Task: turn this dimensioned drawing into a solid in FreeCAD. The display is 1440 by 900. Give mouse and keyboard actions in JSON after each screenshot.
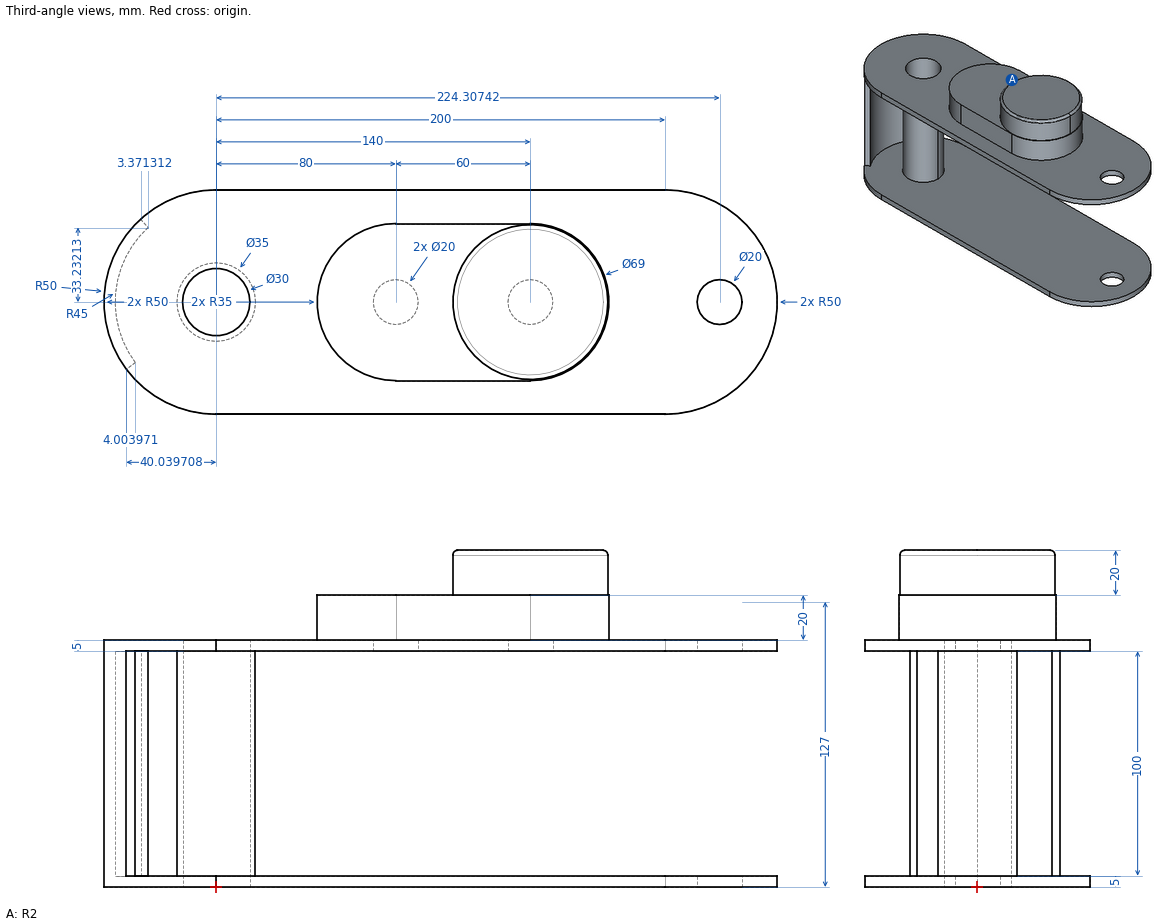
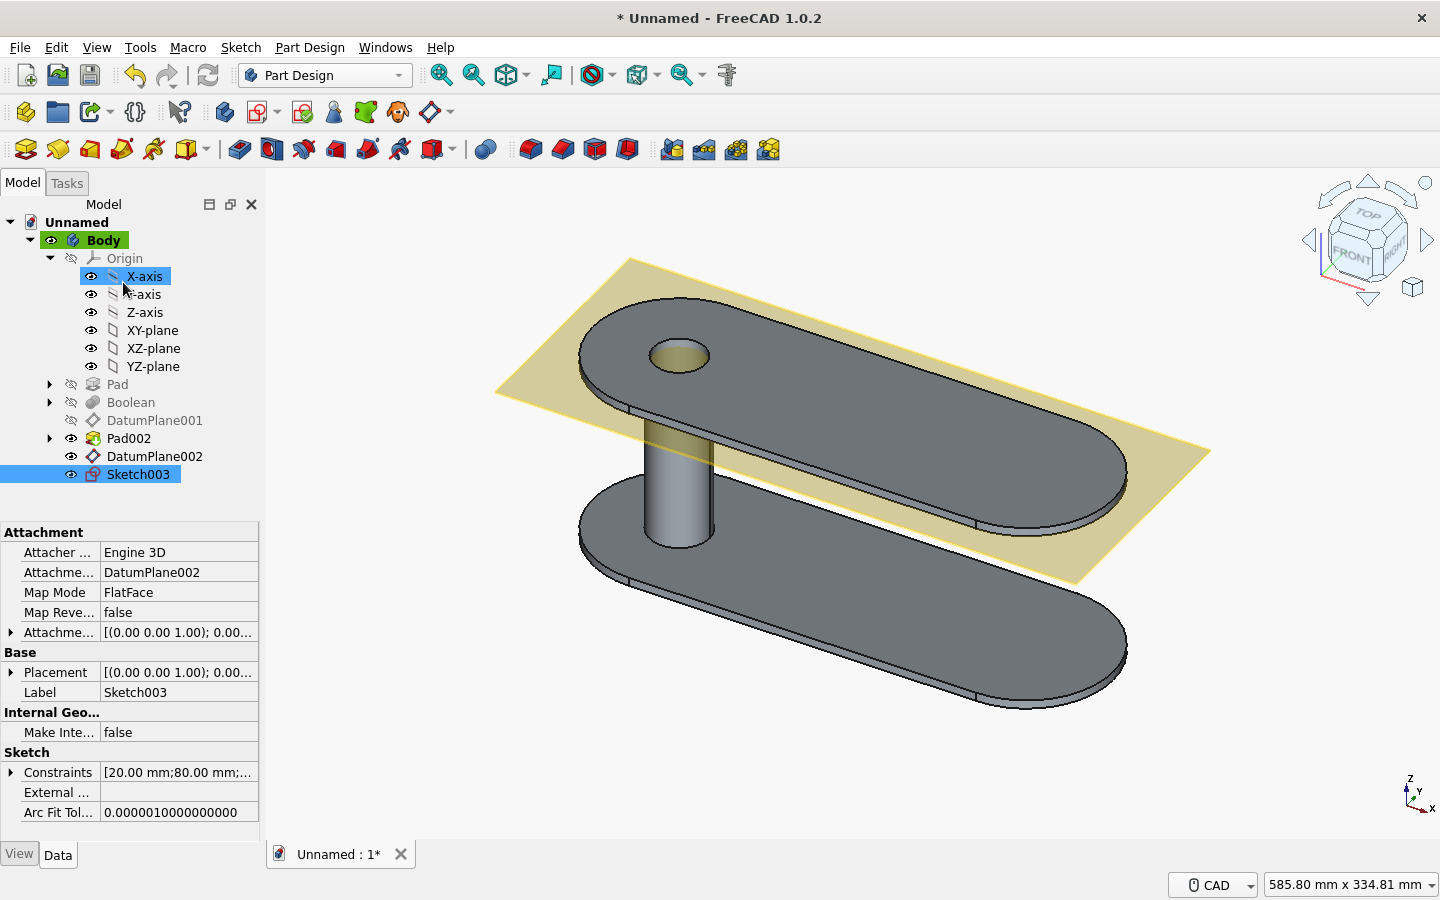
{"action": "left_click", "coordinate": [240, 150]}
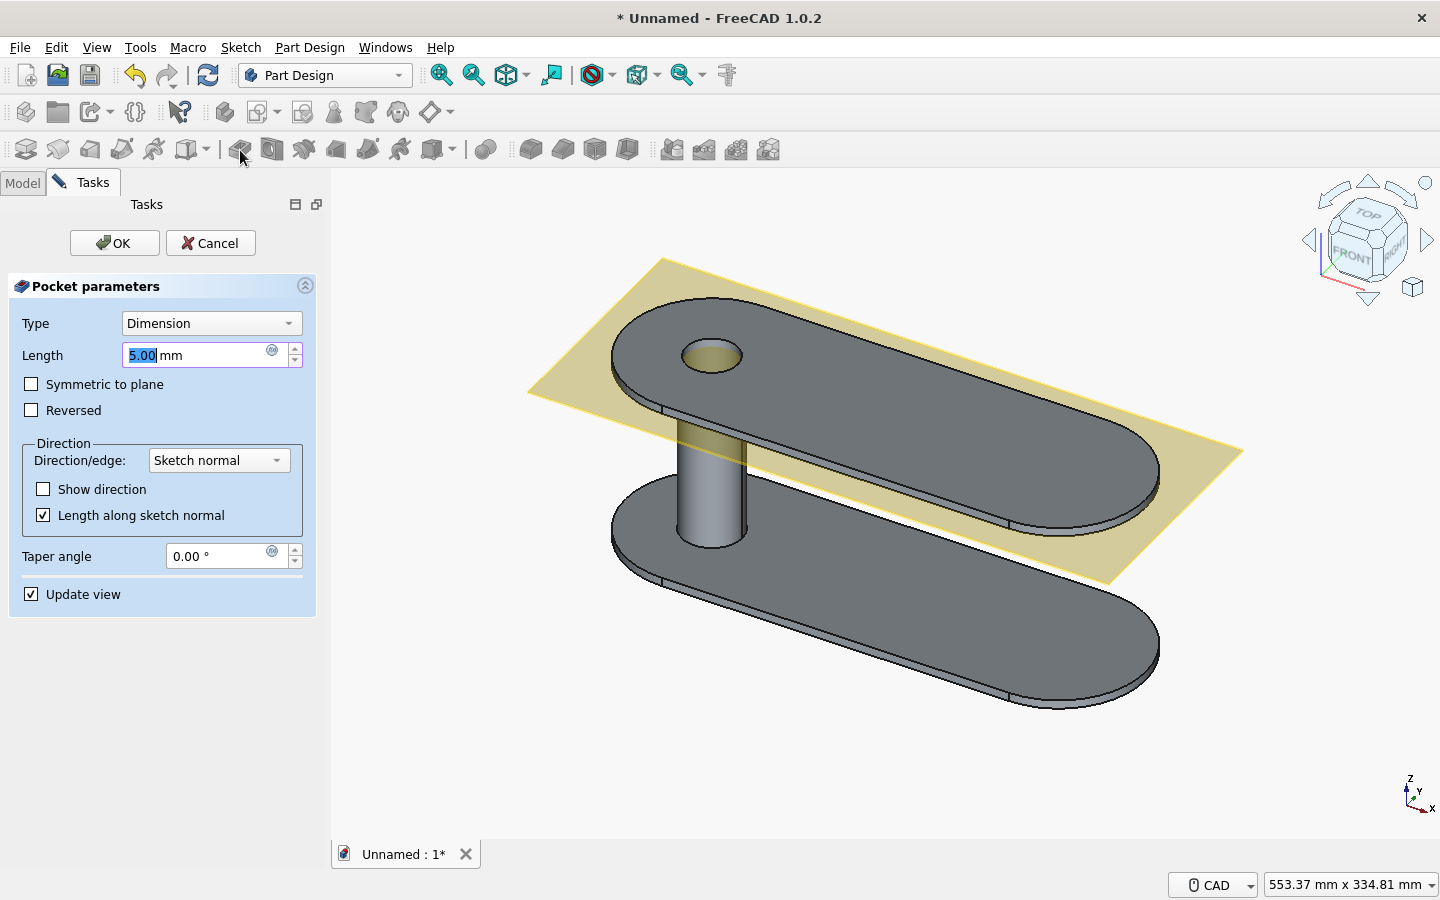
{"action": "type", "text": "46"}
{"action": "key", "text": "Tab"}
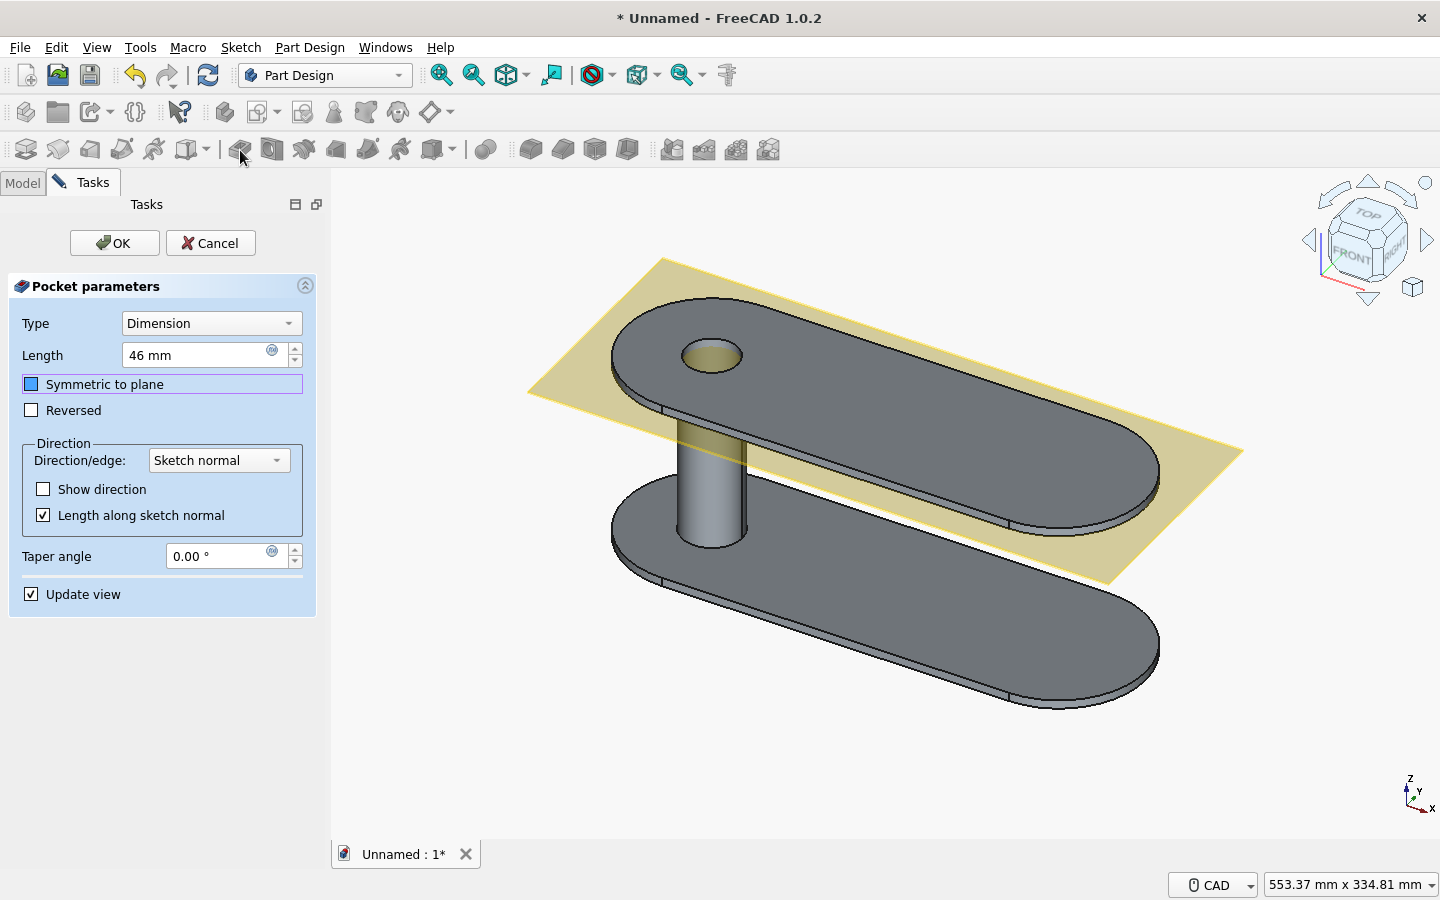
{"action": "left_click", "coordinate": [30, 410]}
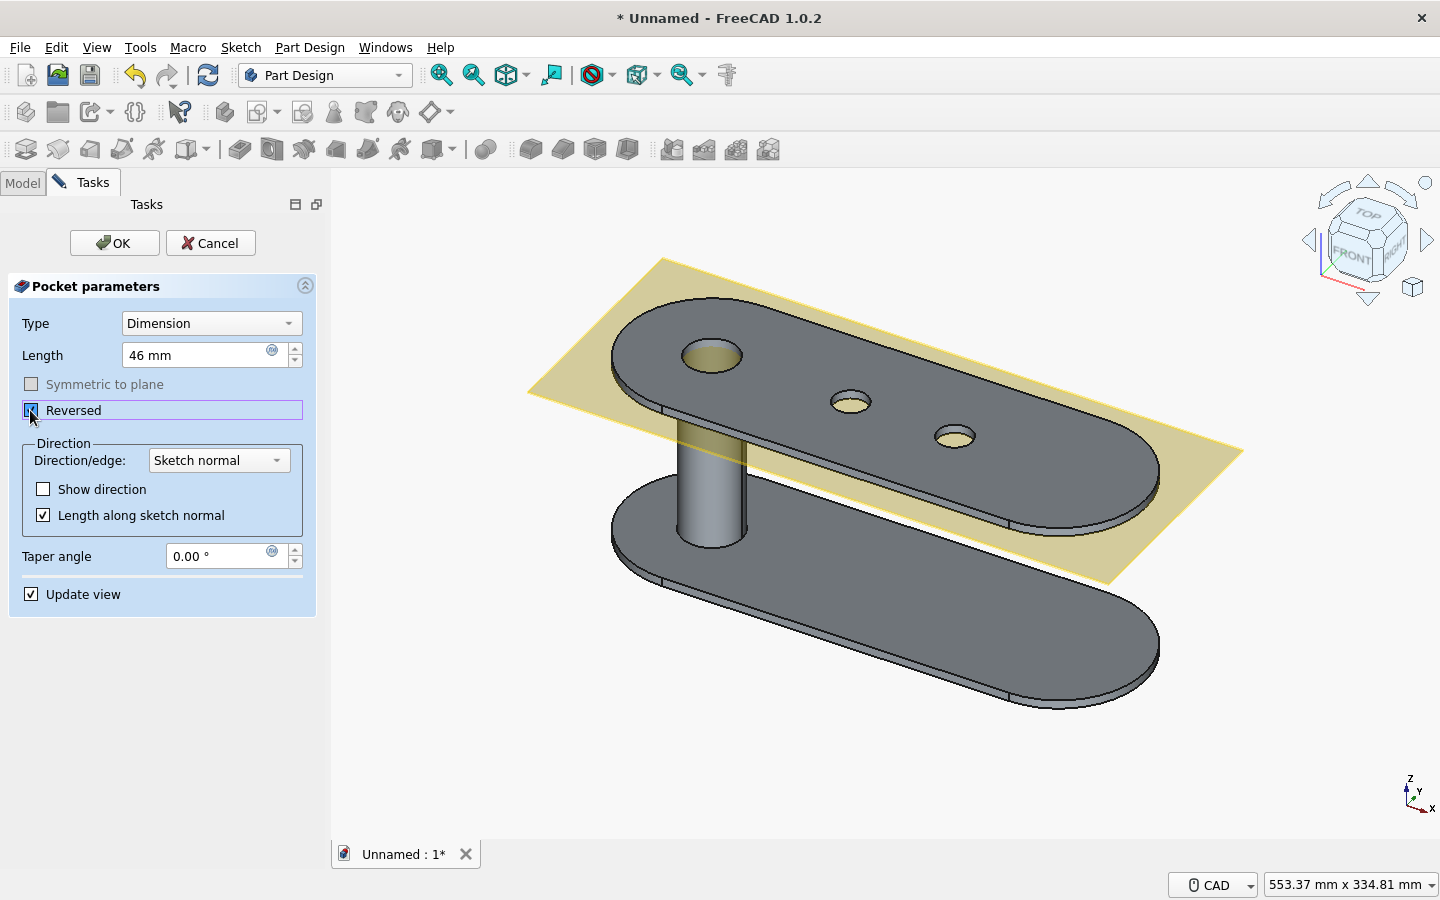
{"action": "left_click", "coordinate": [115, 243]}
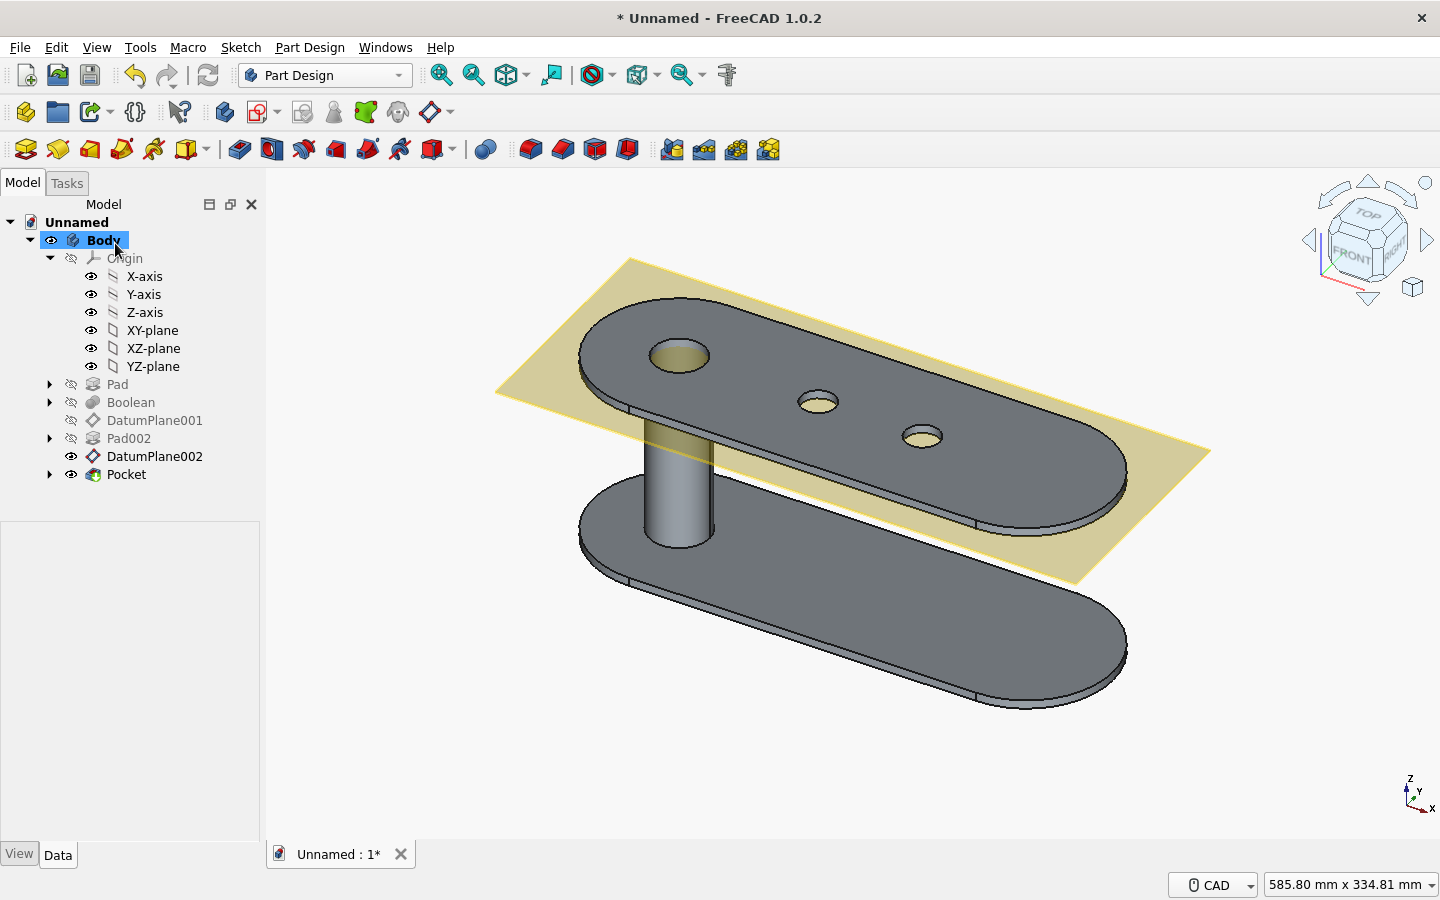
{"action": "left_click", "coordinate": [116, 456]}
{"action": "key", "text": "space"}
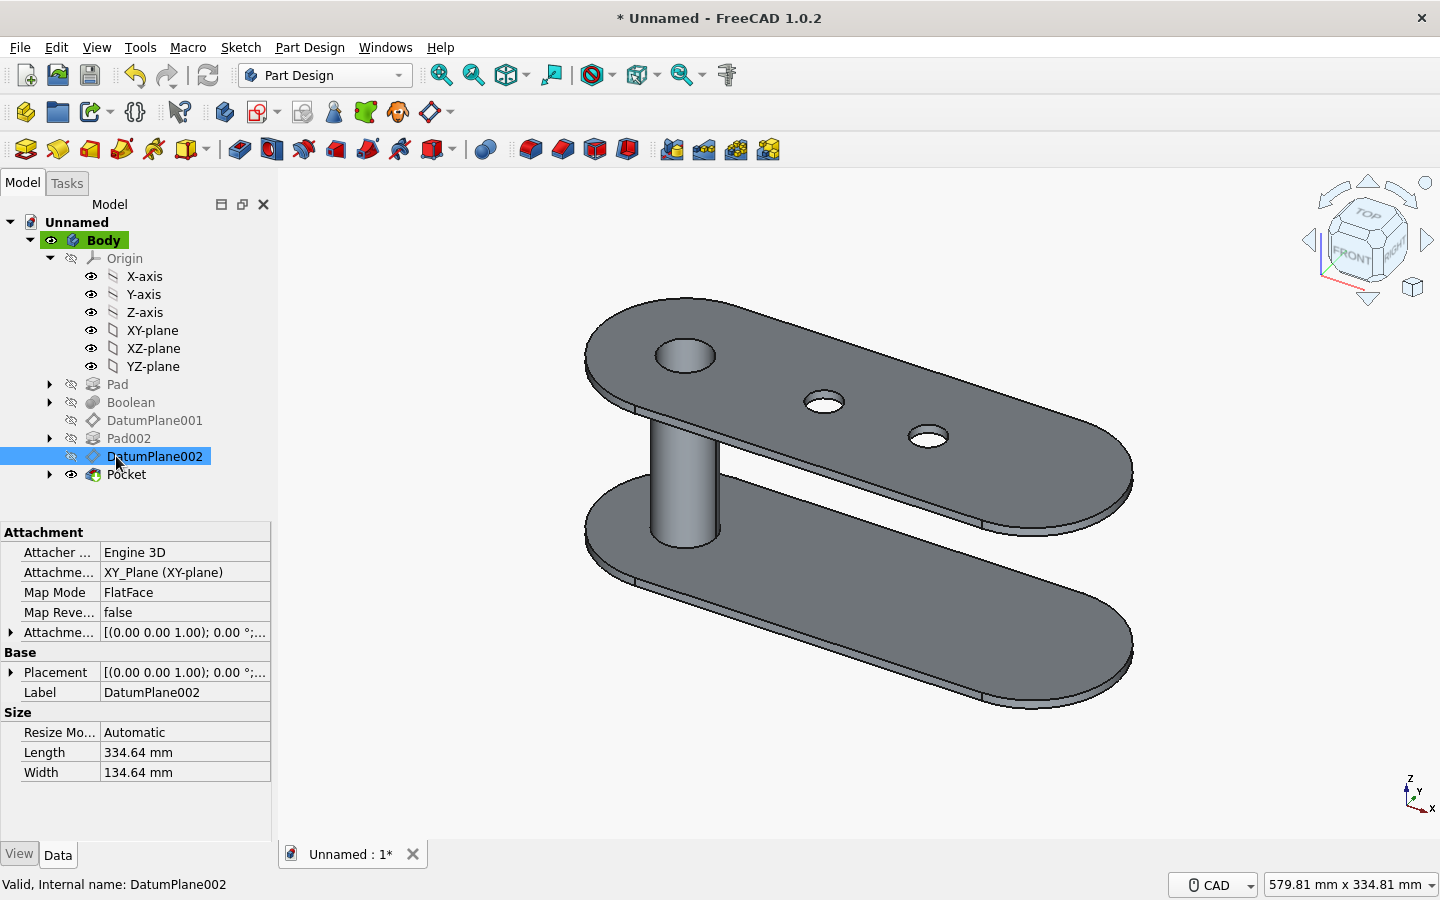
{"action": "left_click", "coordinate": [1008, 461]}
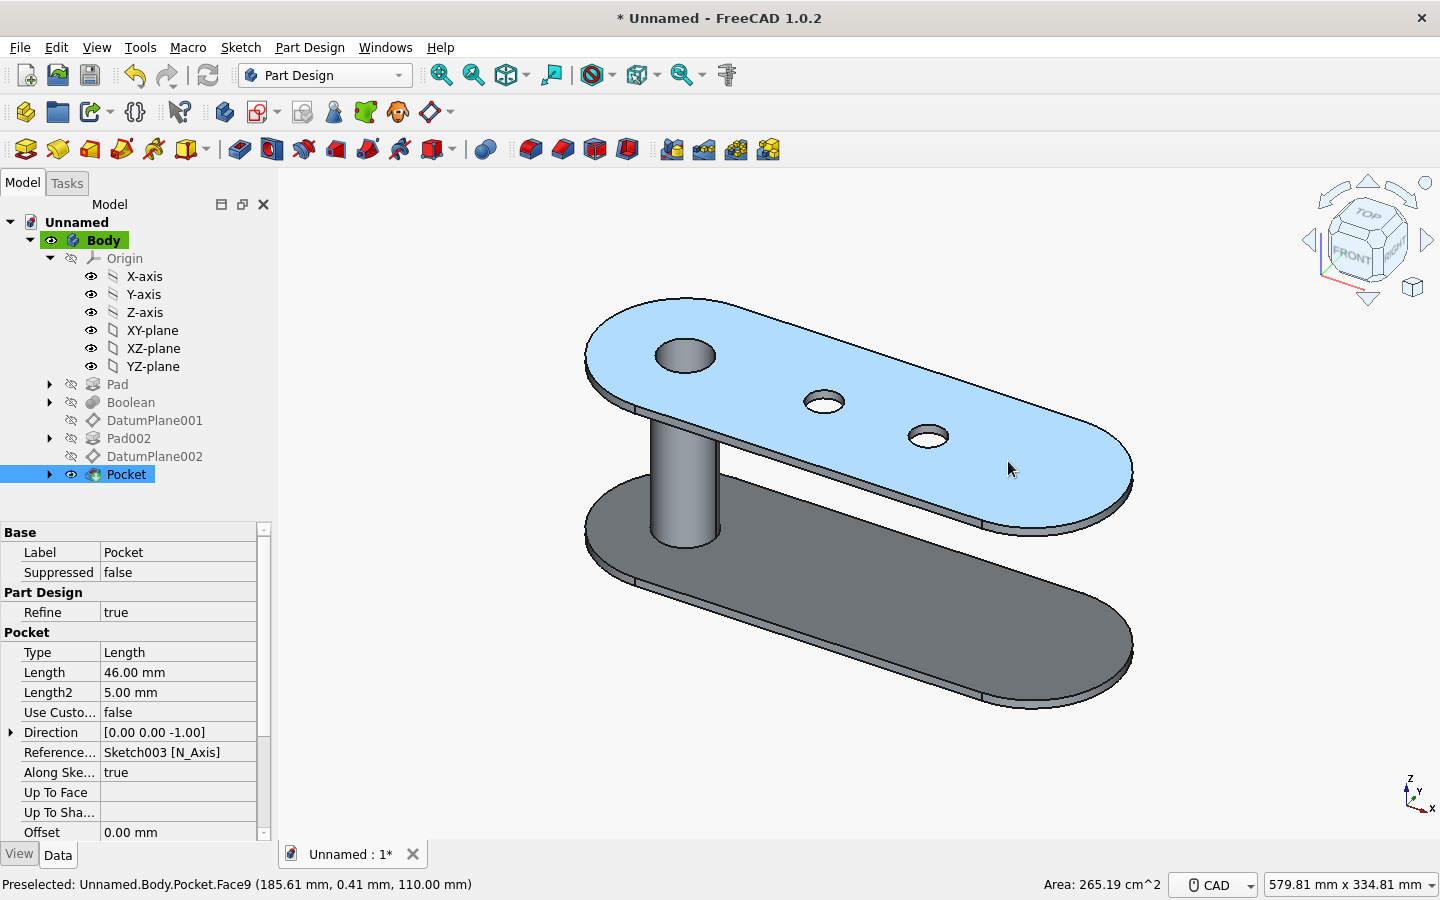
{"action": "left_click", "coordinate": [258, 112]}